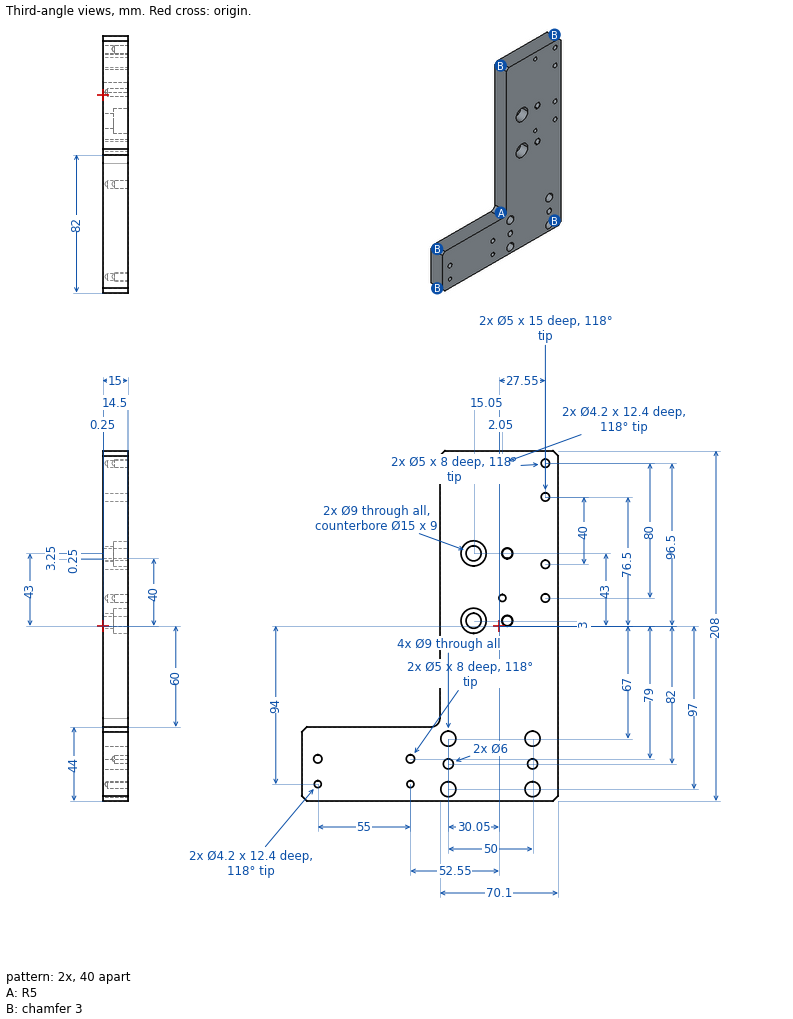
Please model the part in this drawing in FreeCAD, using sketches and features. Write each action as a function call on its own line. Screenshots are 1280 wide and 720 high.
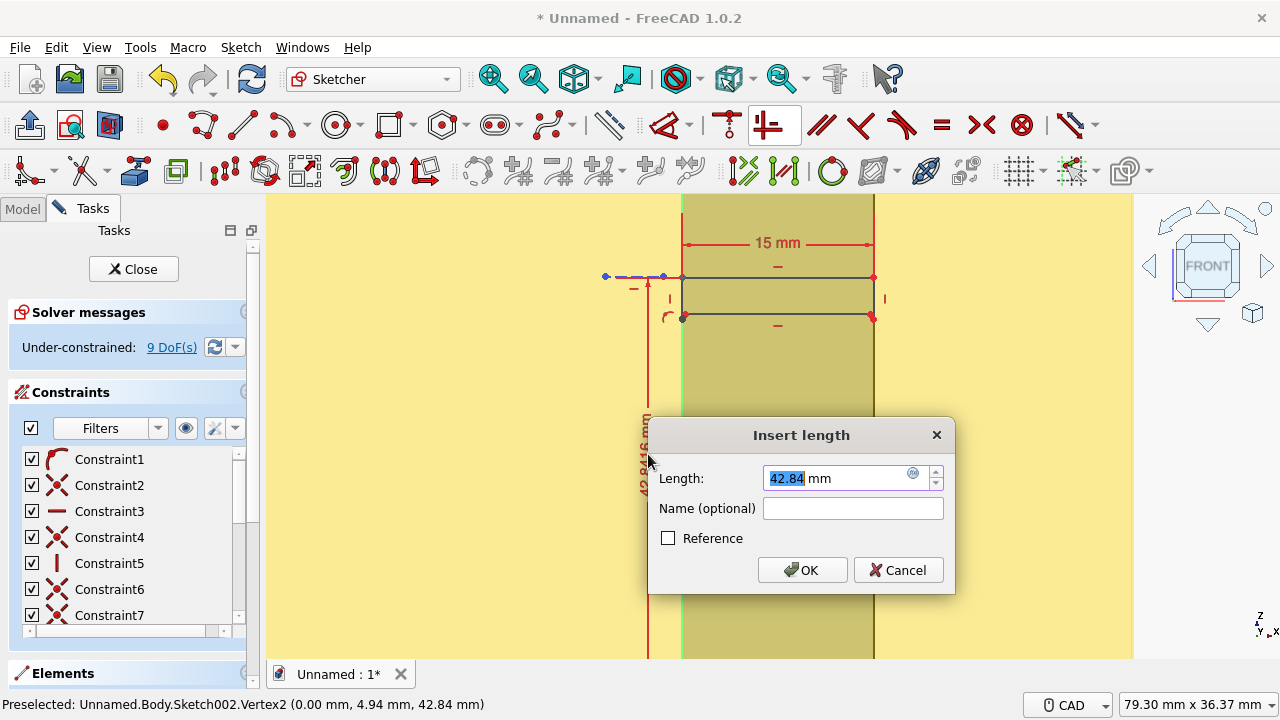
text(43)
key(Return)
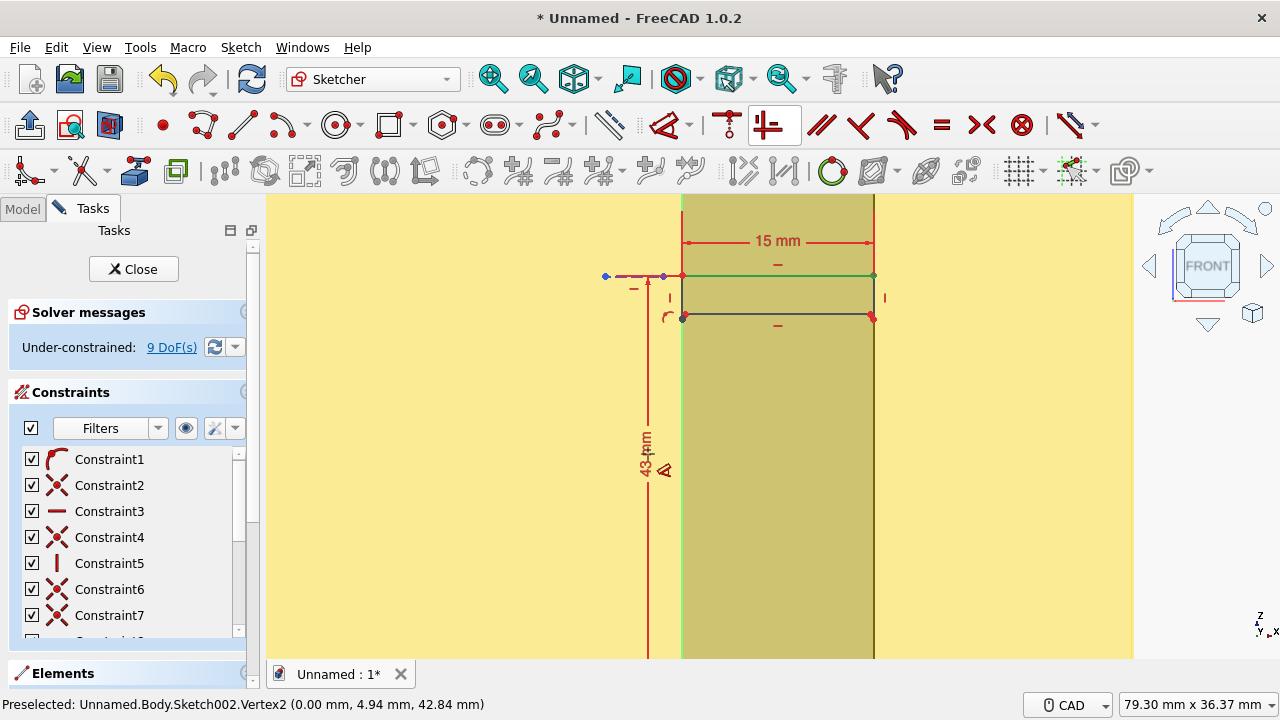
scroll(871, 314, up, 4)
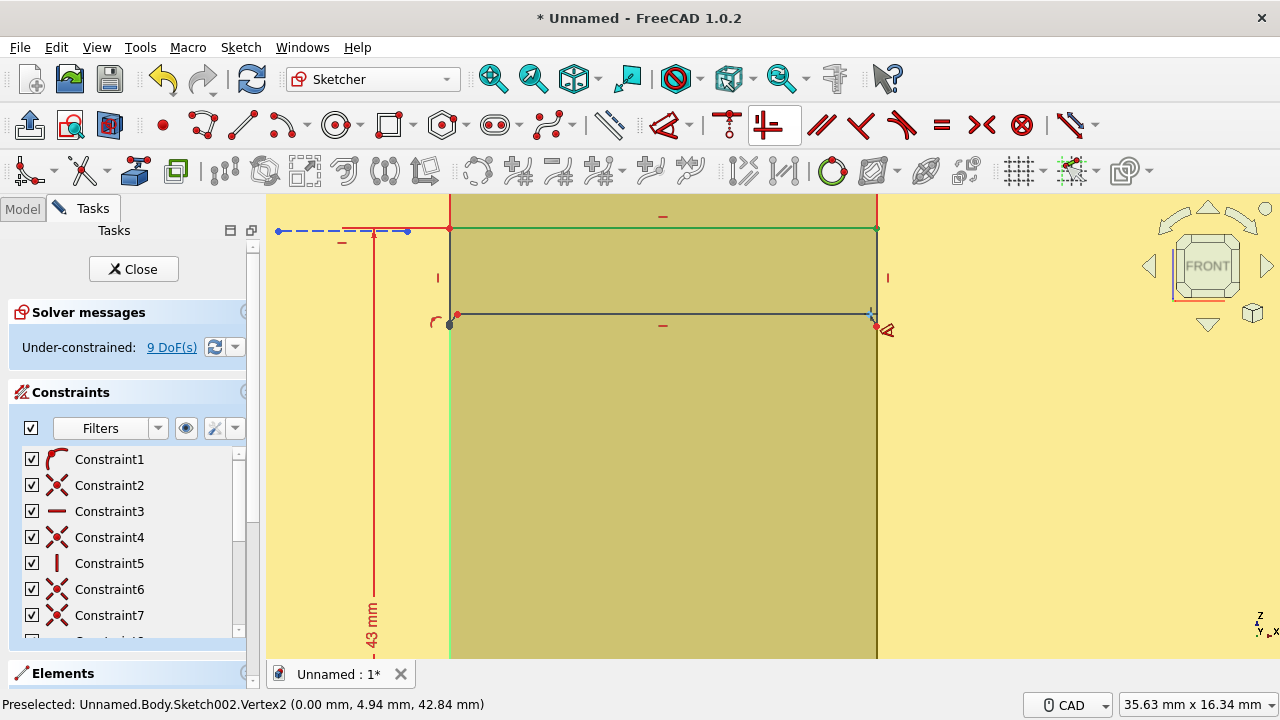
click(870, 314)
click(904, 473)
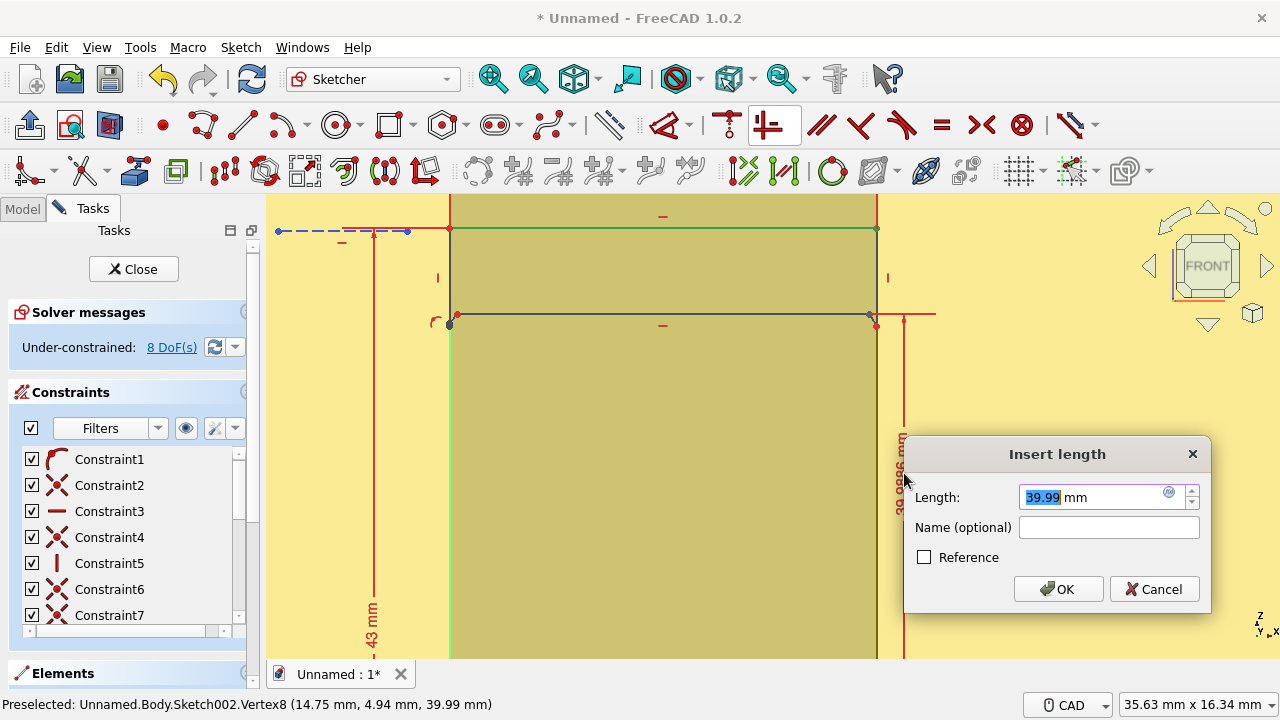
text(40)
key(Return)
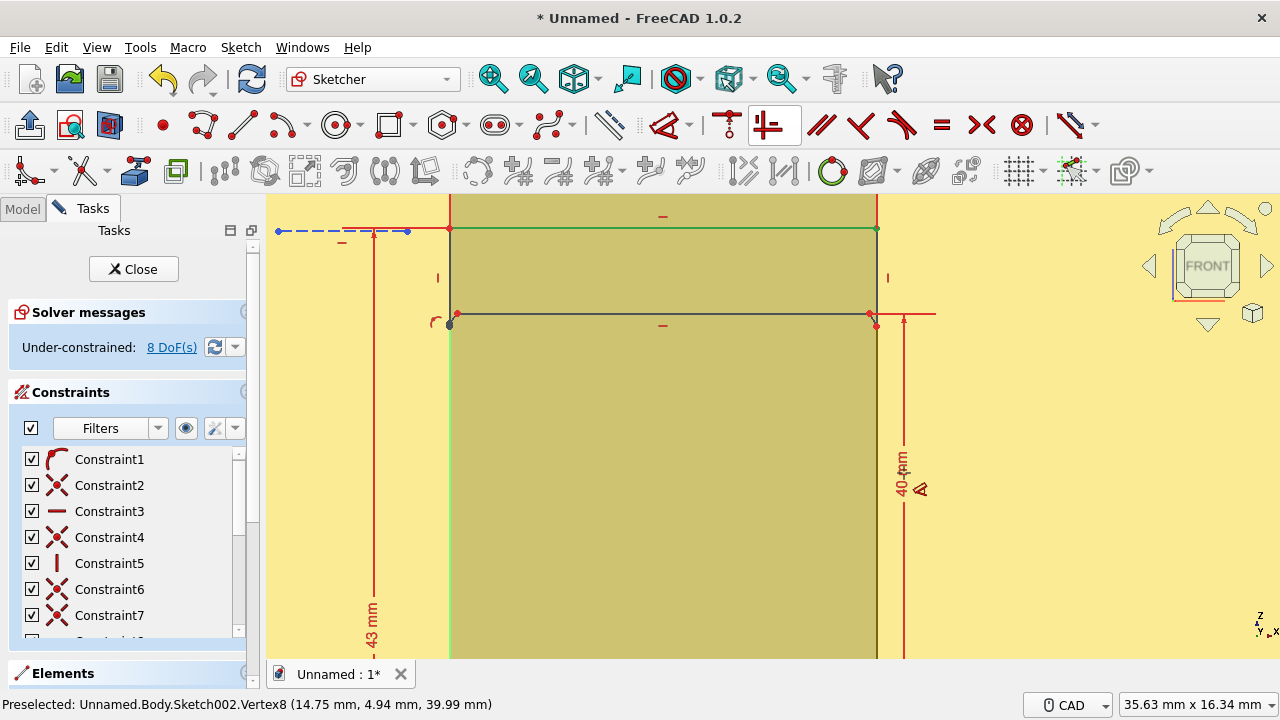
scroll(746, 291, down, 7)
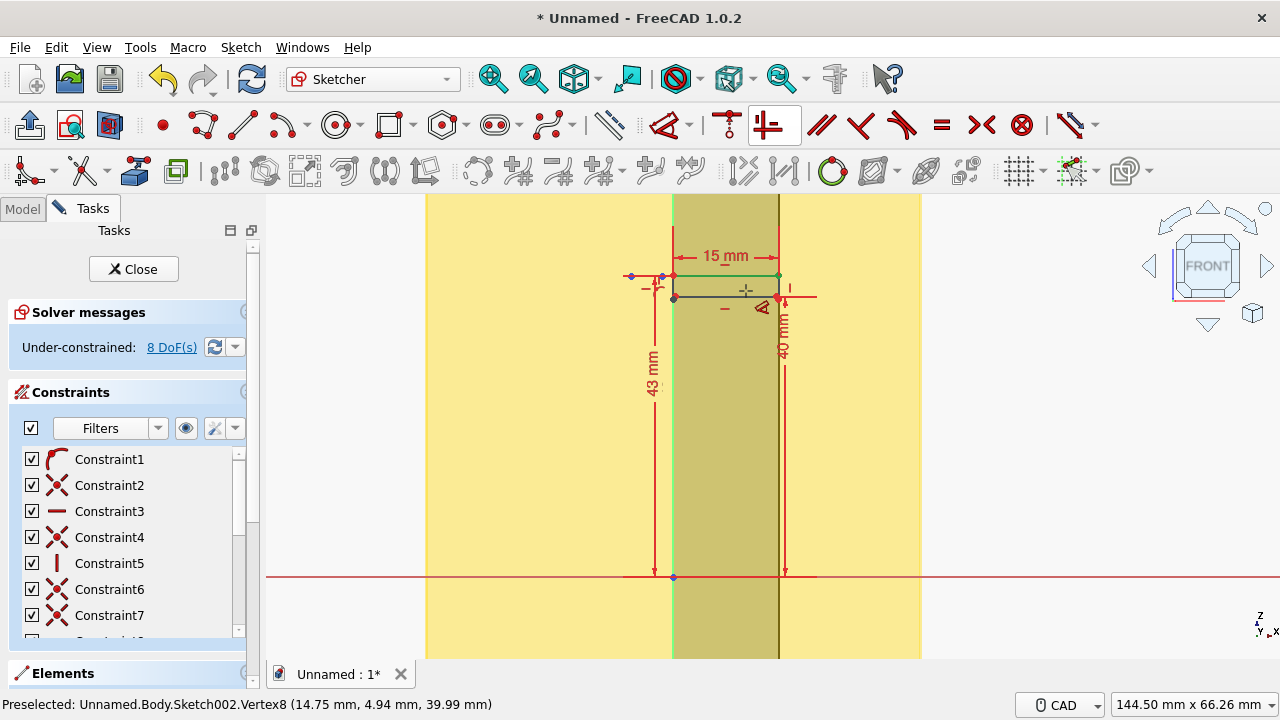
click(663, 276)
click(629, 427)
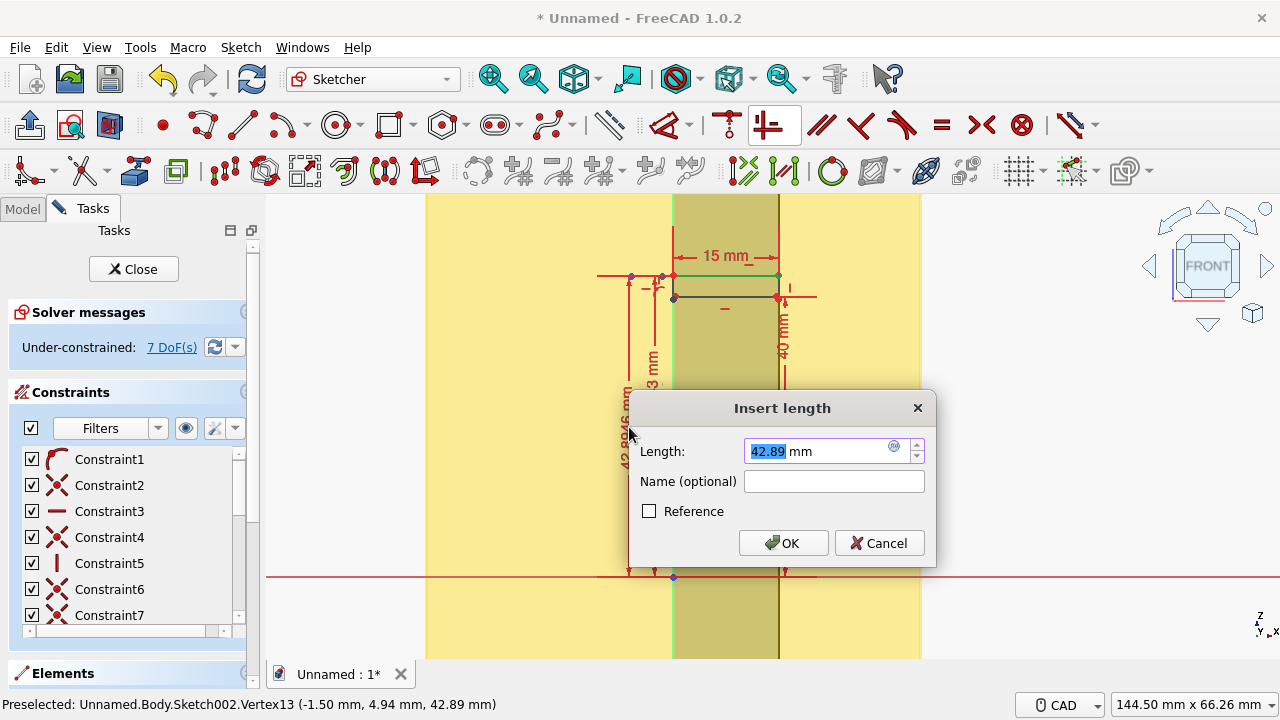
text(43)
key(Return)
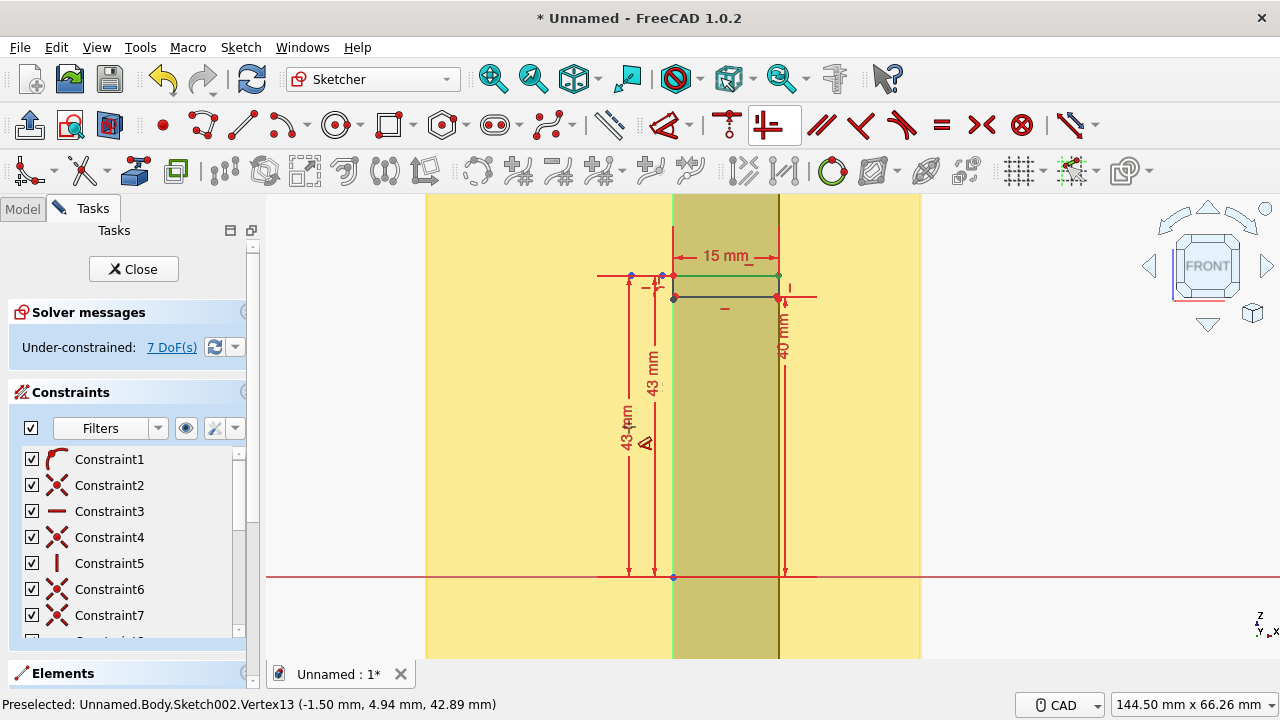
scroll(673, 285, up, 3)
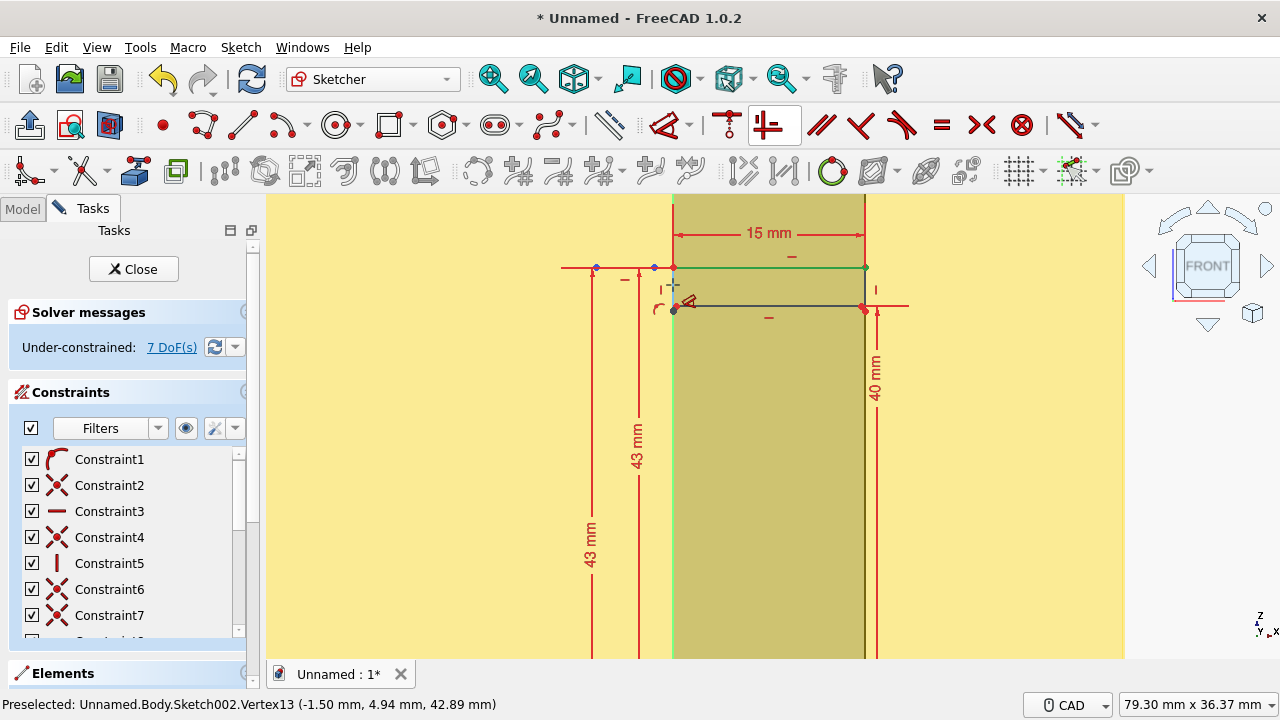
click(673, 285)
click(639, 290)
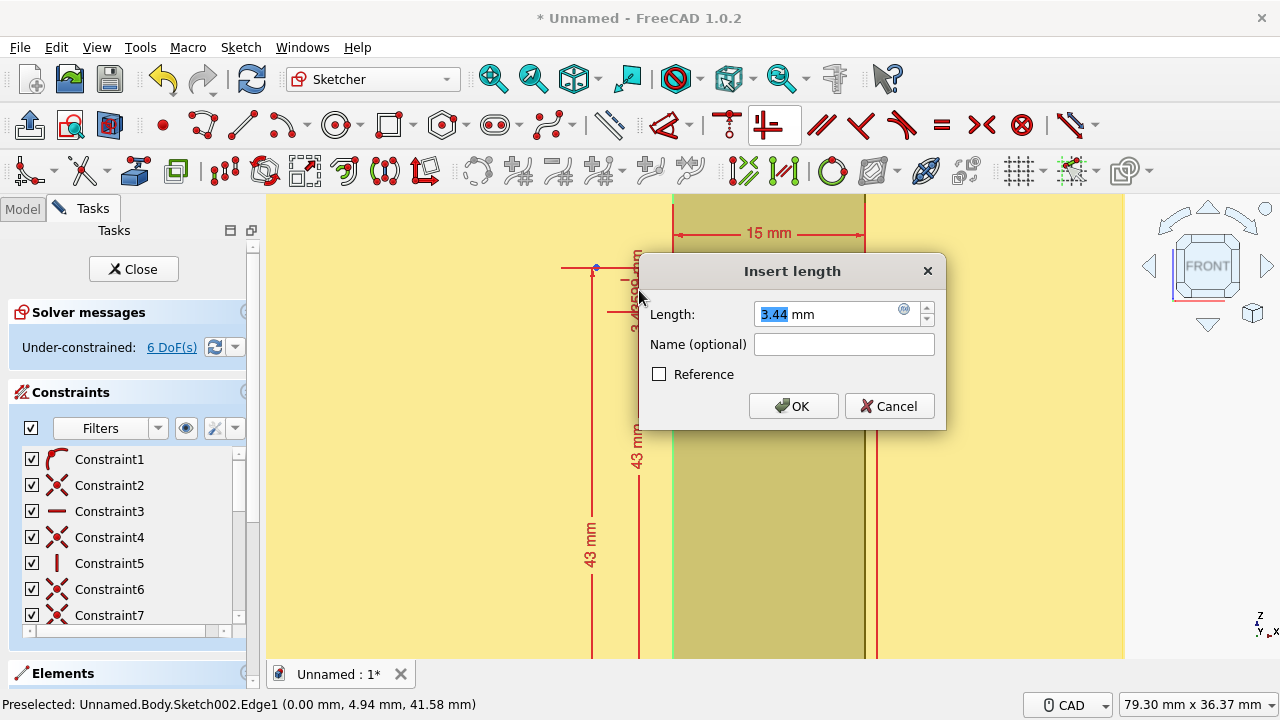
text(3.25)
key(Return)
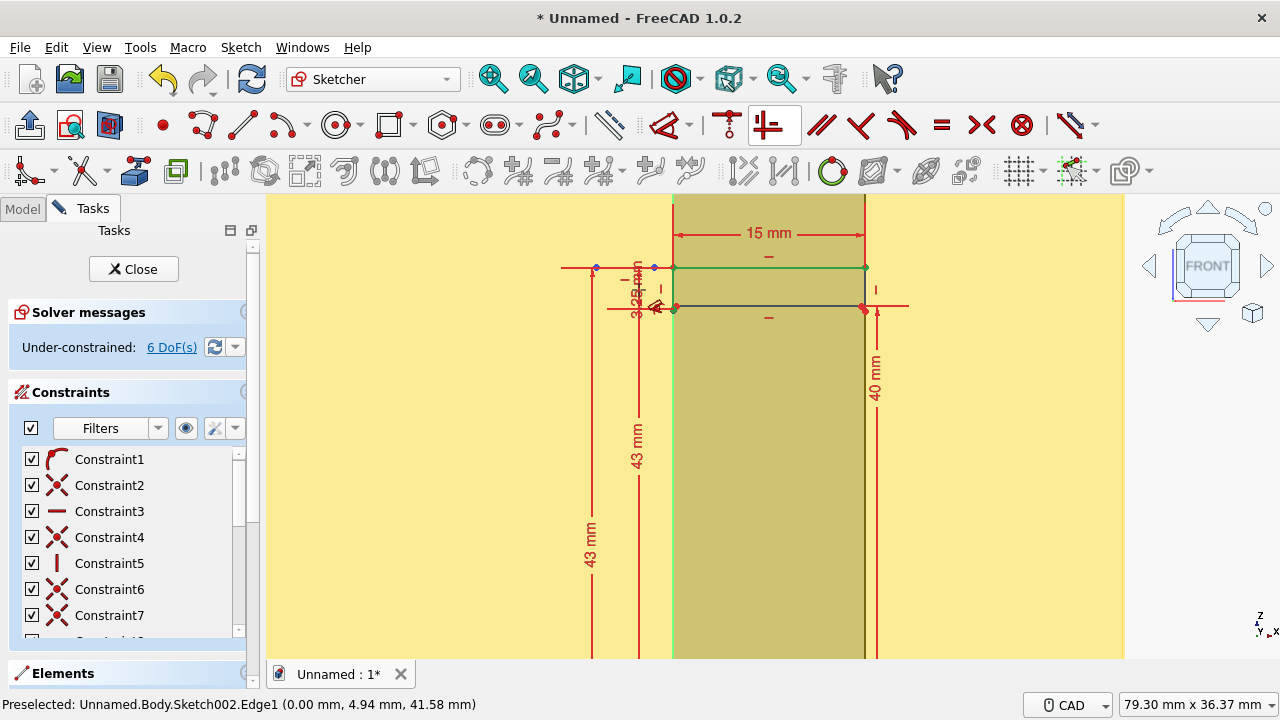
click(865, 281)
click(899, 290)